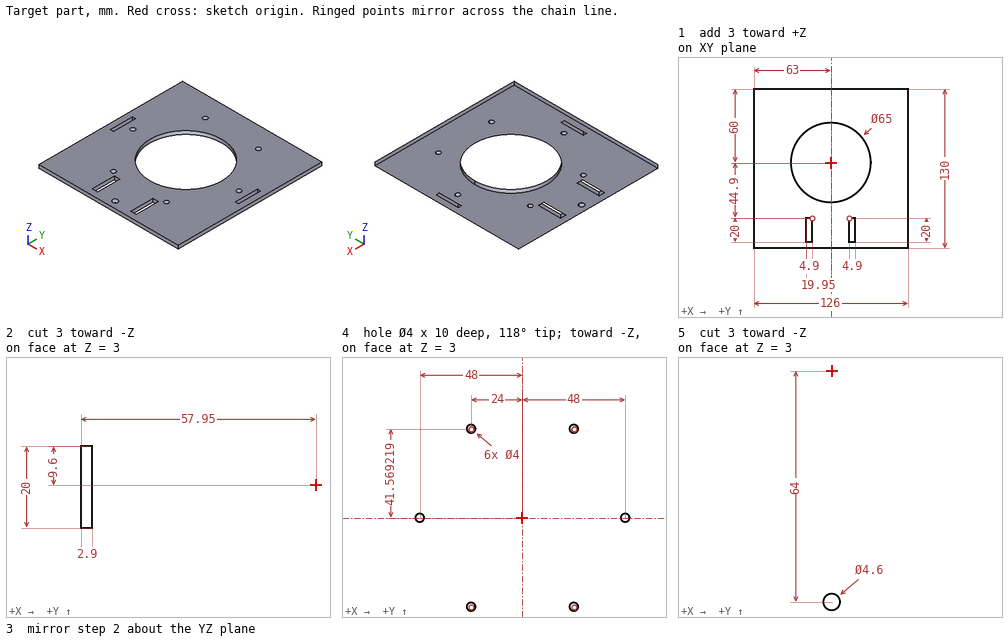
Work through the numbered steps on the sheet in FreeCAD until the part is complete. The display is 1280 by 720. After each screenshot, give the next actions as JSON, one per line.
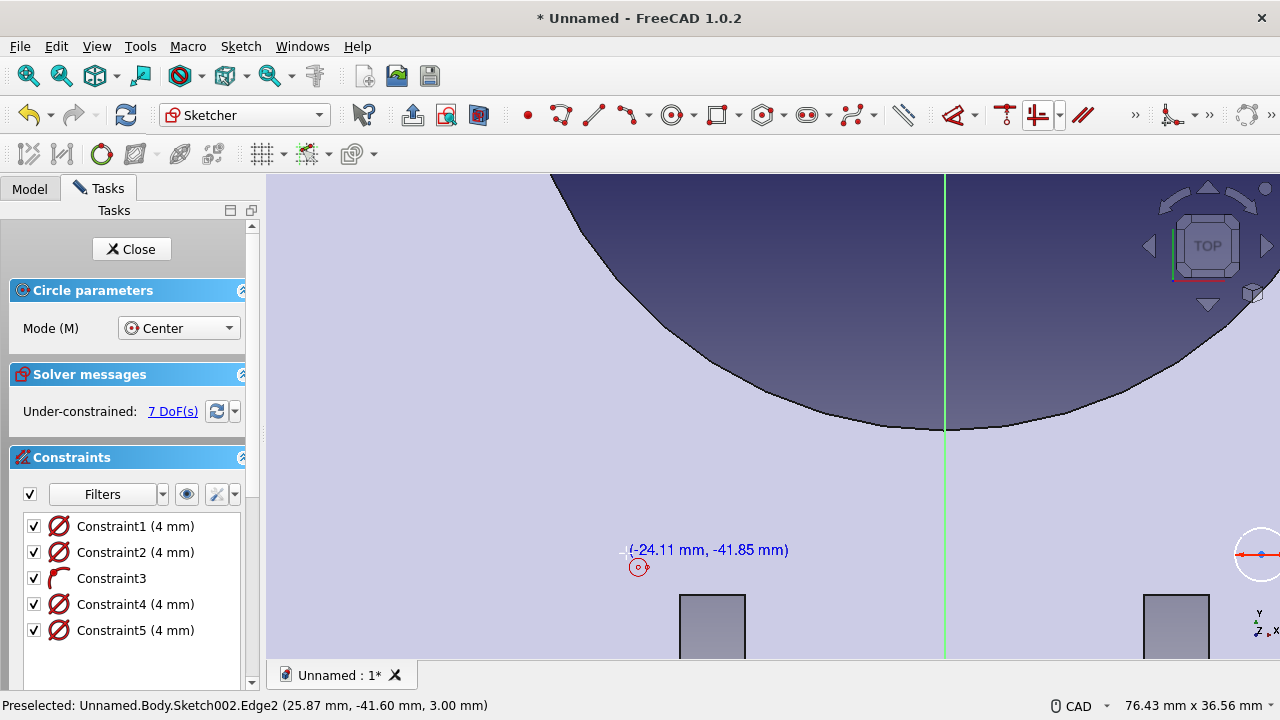
{"action": "scroll", "coordinate": [626, 553], "scroll_direction": "down", "scroll_amount": 7}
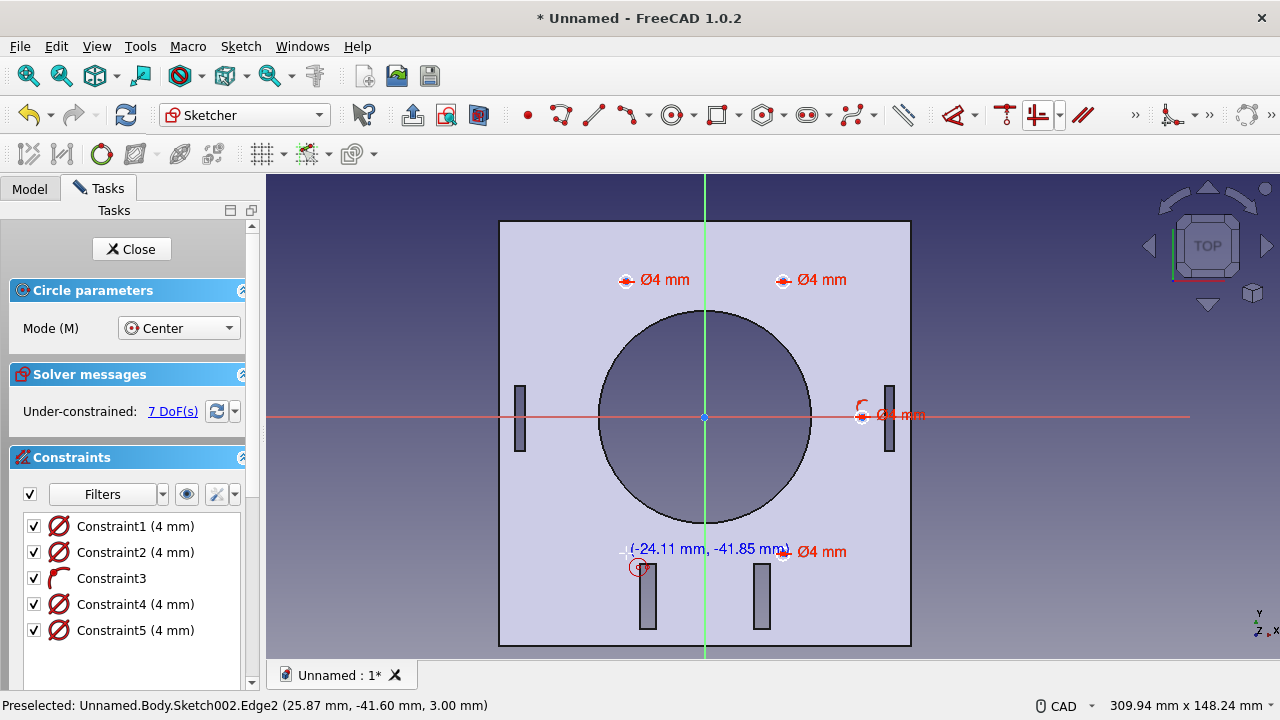
{"action": "left_click", "coordinate": [626, 553]}
{"action": "mouse_move", "coordinate": [631, 548]}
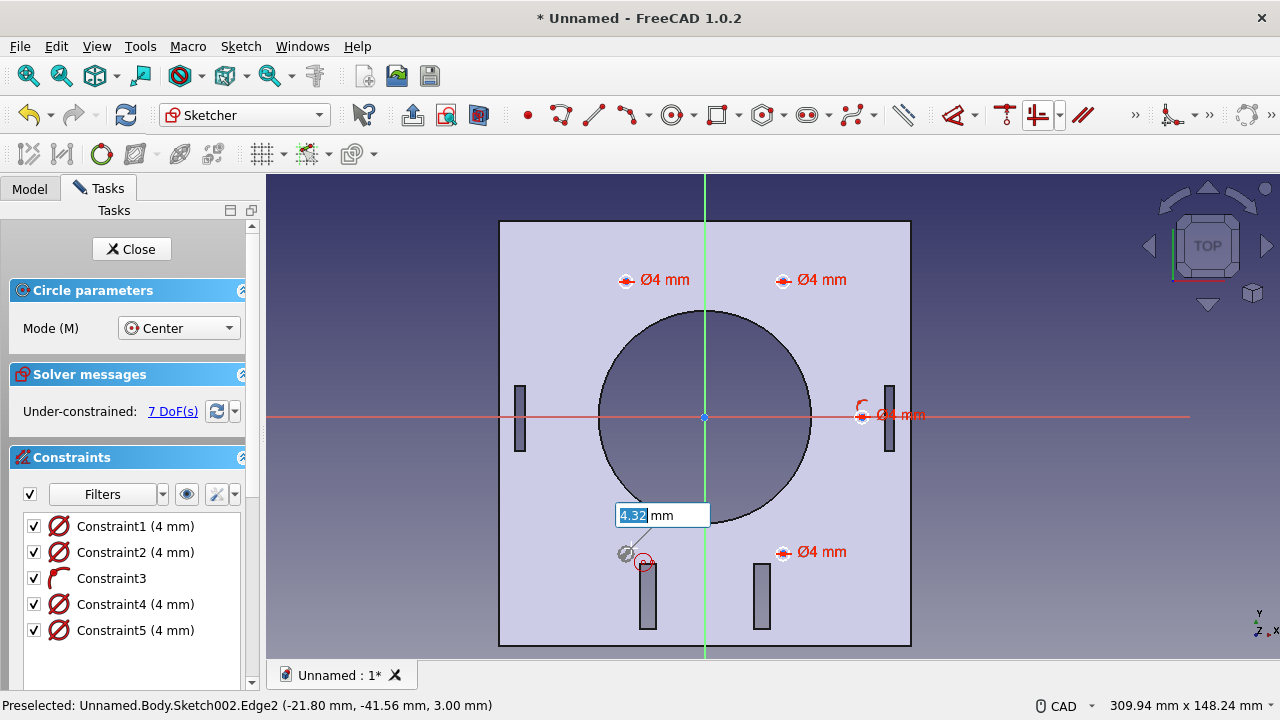
{"action": "type", "text": "4"}
{"action": "key", "text": "Return"}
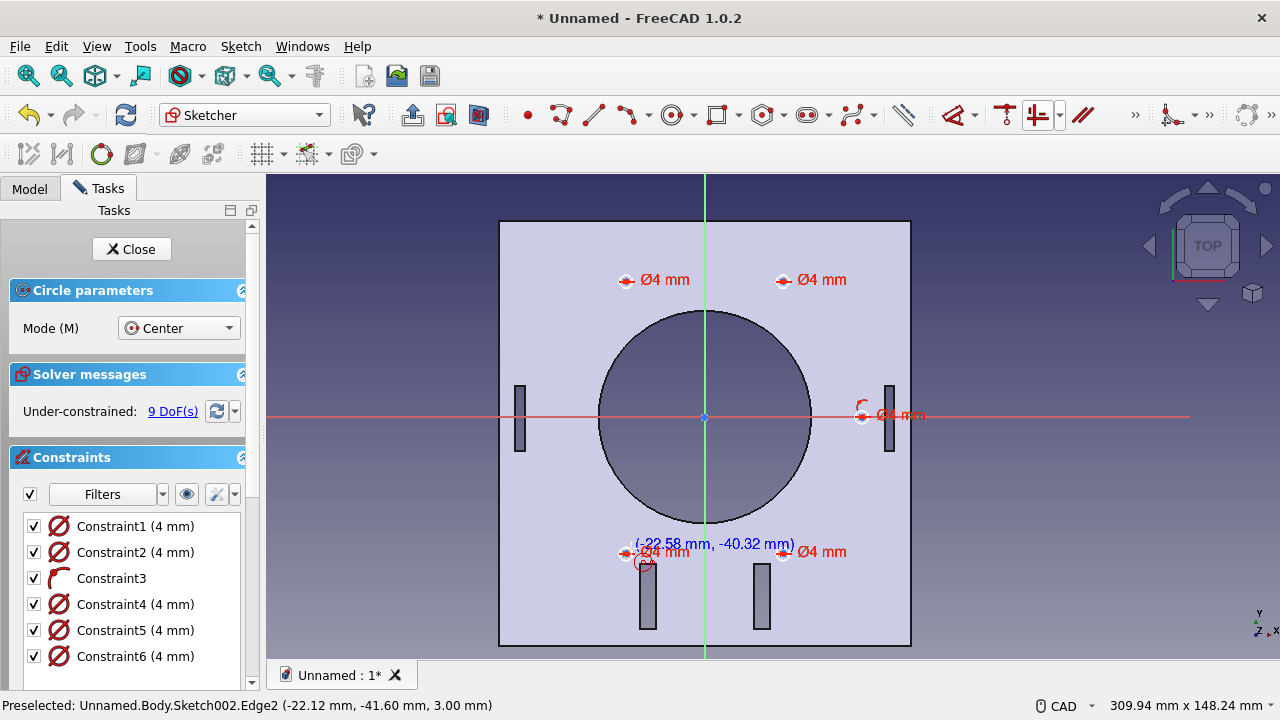
{"action": "scroll", "coordinate": [548, 417], "scroll_direction": "up", "scroll_amount": 7}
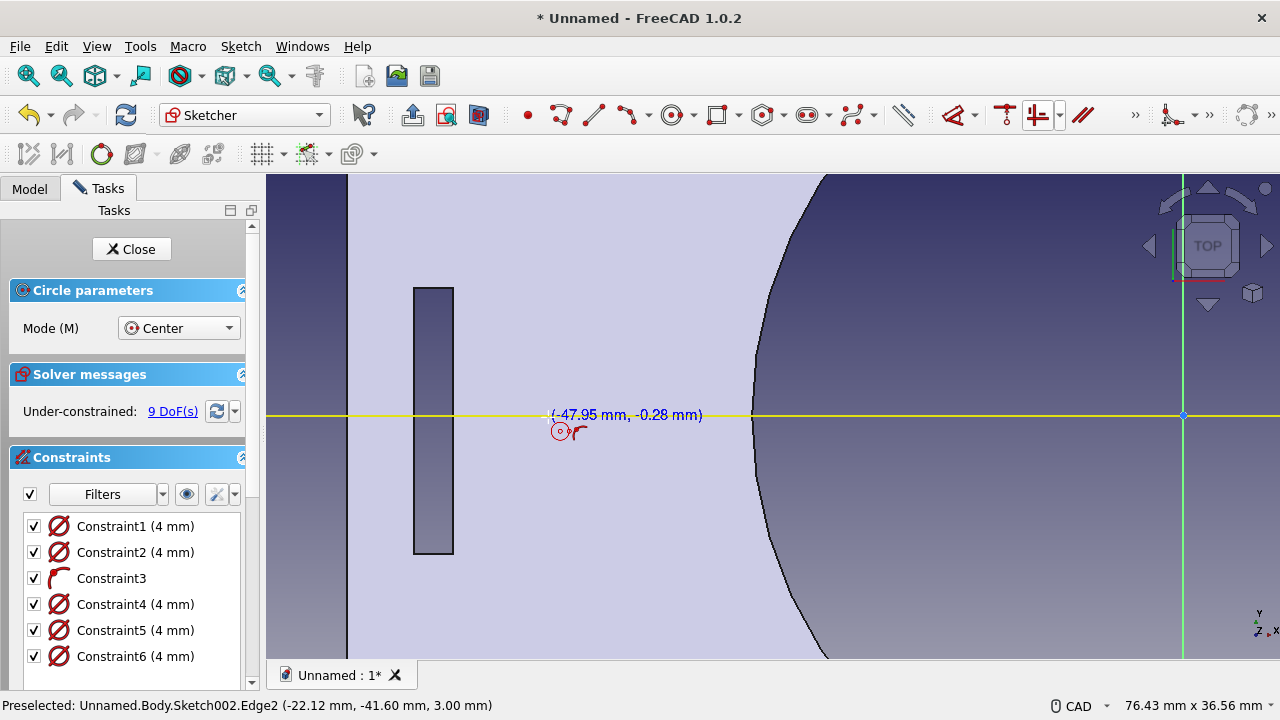
{"action": "scroll", "coordinate": [548, 417], "scroll_direction": "down", "scroll_amount": 7}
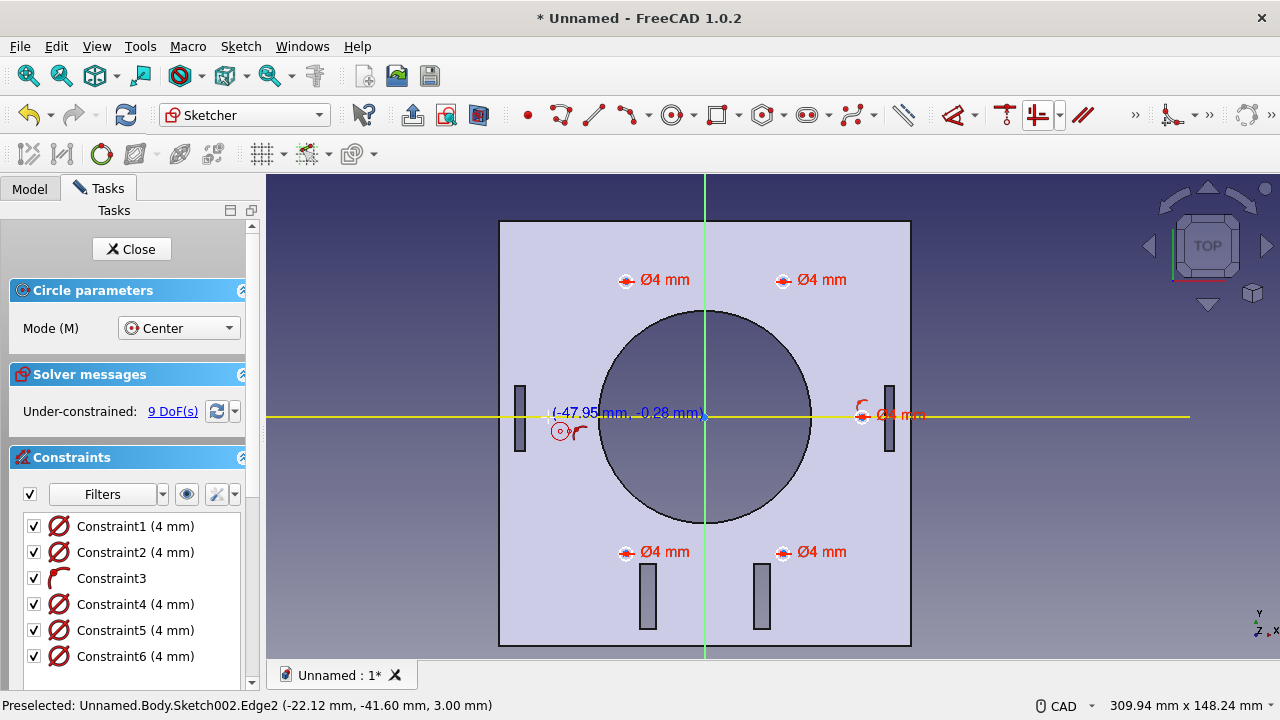
{"action": "left_click", "coordinate": [548, 417]}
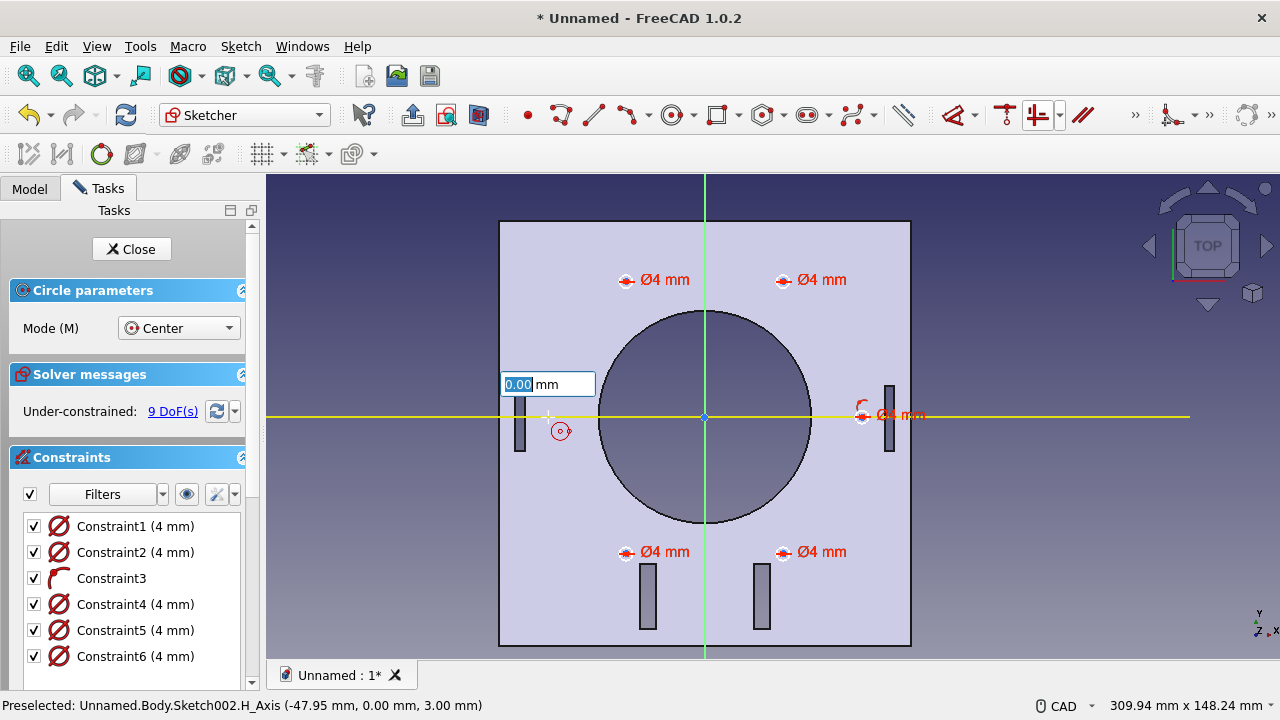
{"action": "scroll", "coordinate": [546, 423], "scroll_direction": "up", "scroll_amount": 5}
{"action": "mouse_move", "coordinate": [544, 423]}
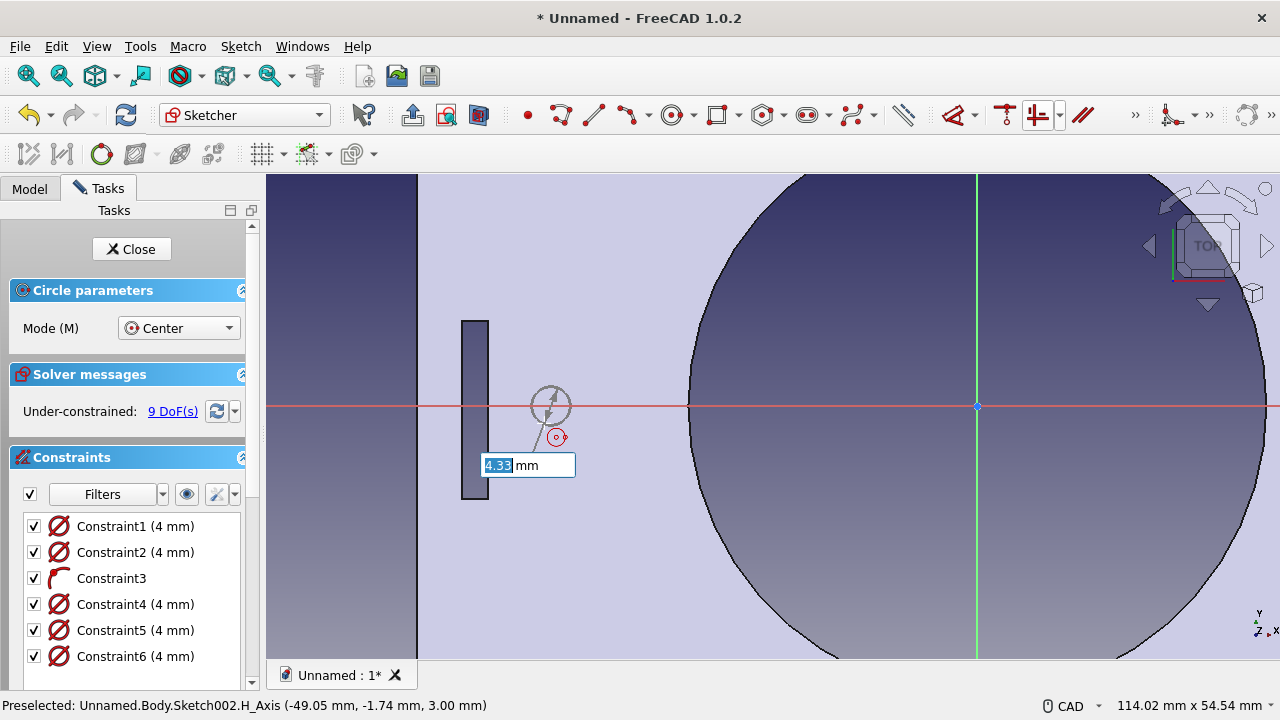
{"action": "type", "text": "4"}
{"action": "key", "text": "Return"}
{"action": "key", "text": "Escape"}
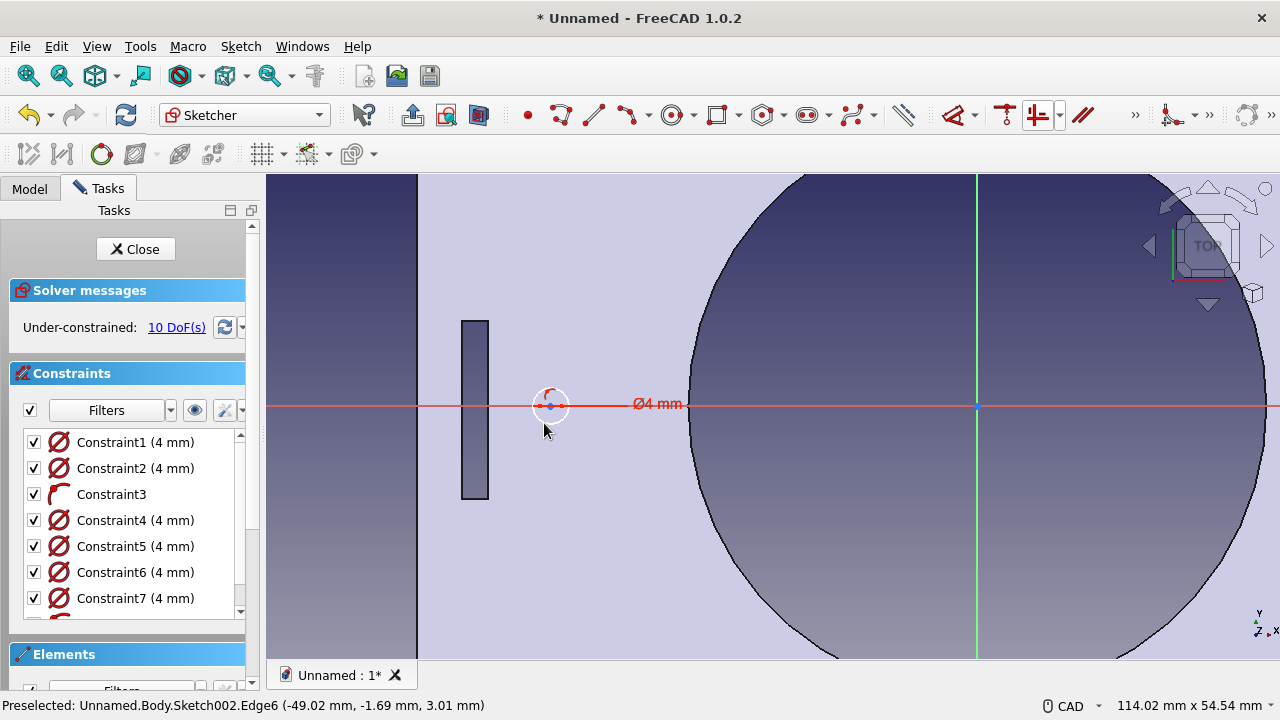
{"action": "scroll", "coordinate": [546, 423], "scroll_direction": "down", "scroll_amount": 5}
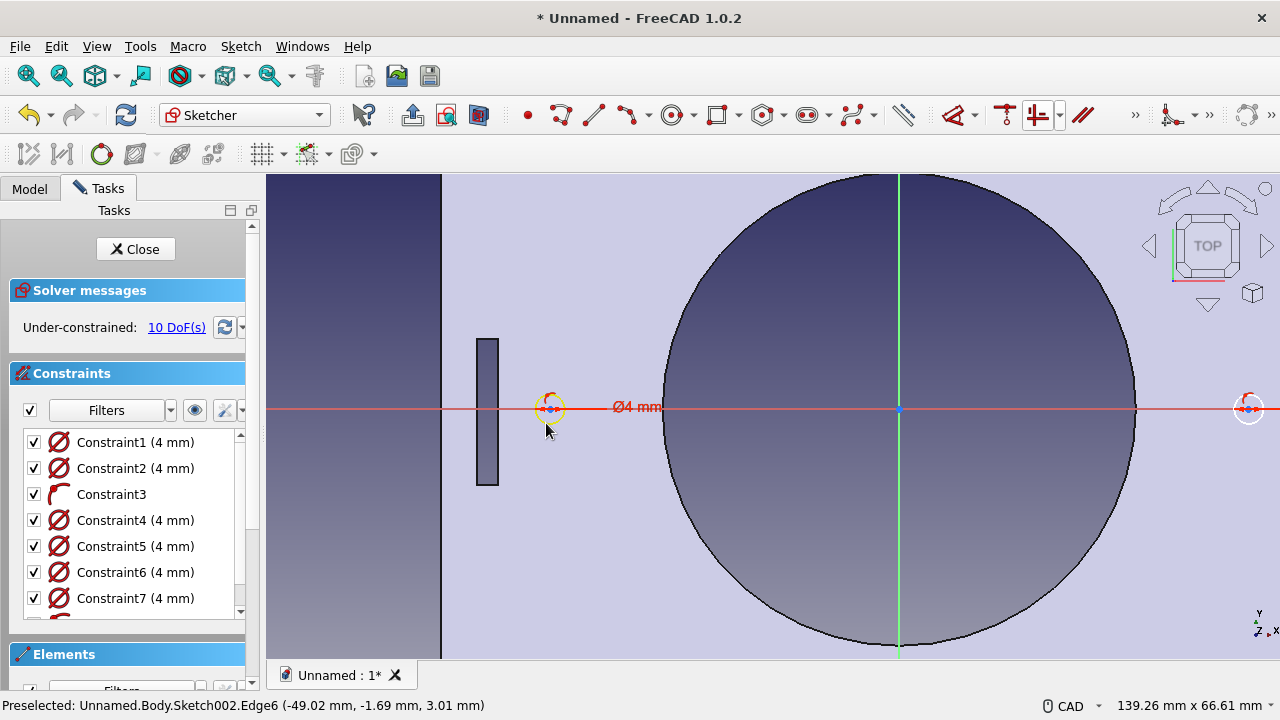
{"action": "left_click", "coordinate": [626, 282]}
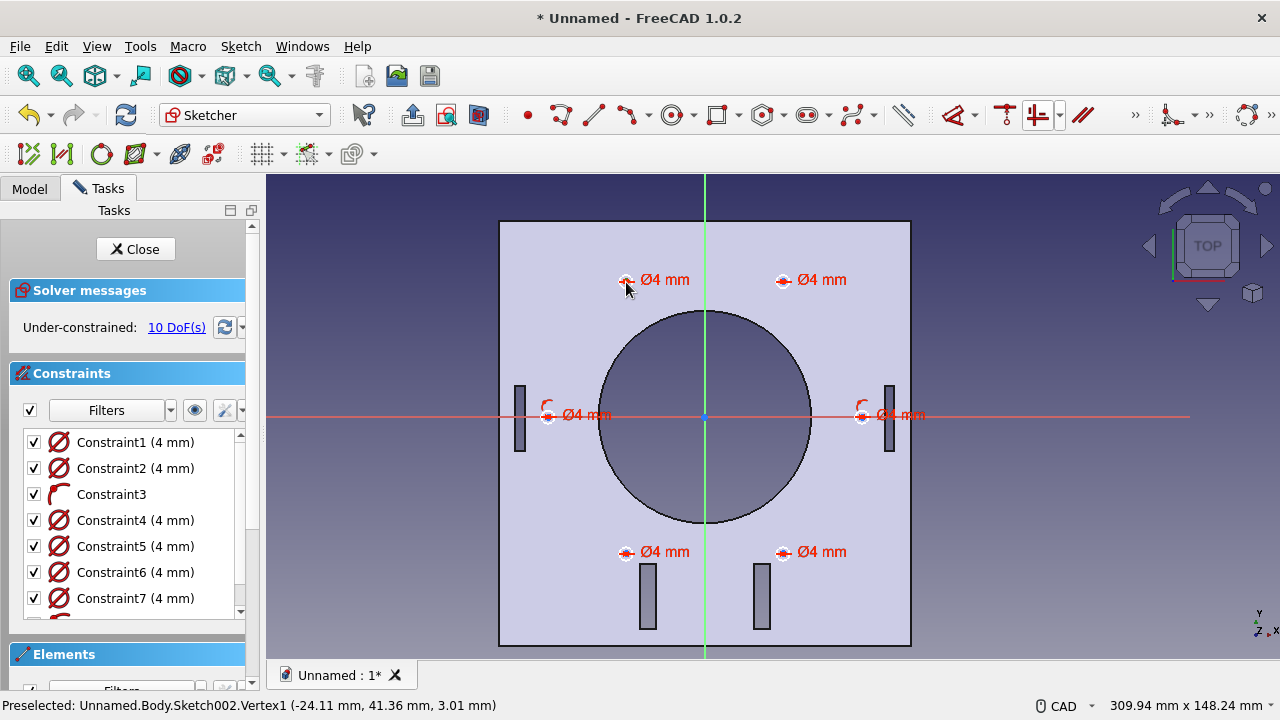
{"action": "left_click", "coordinate": [783, 282]}